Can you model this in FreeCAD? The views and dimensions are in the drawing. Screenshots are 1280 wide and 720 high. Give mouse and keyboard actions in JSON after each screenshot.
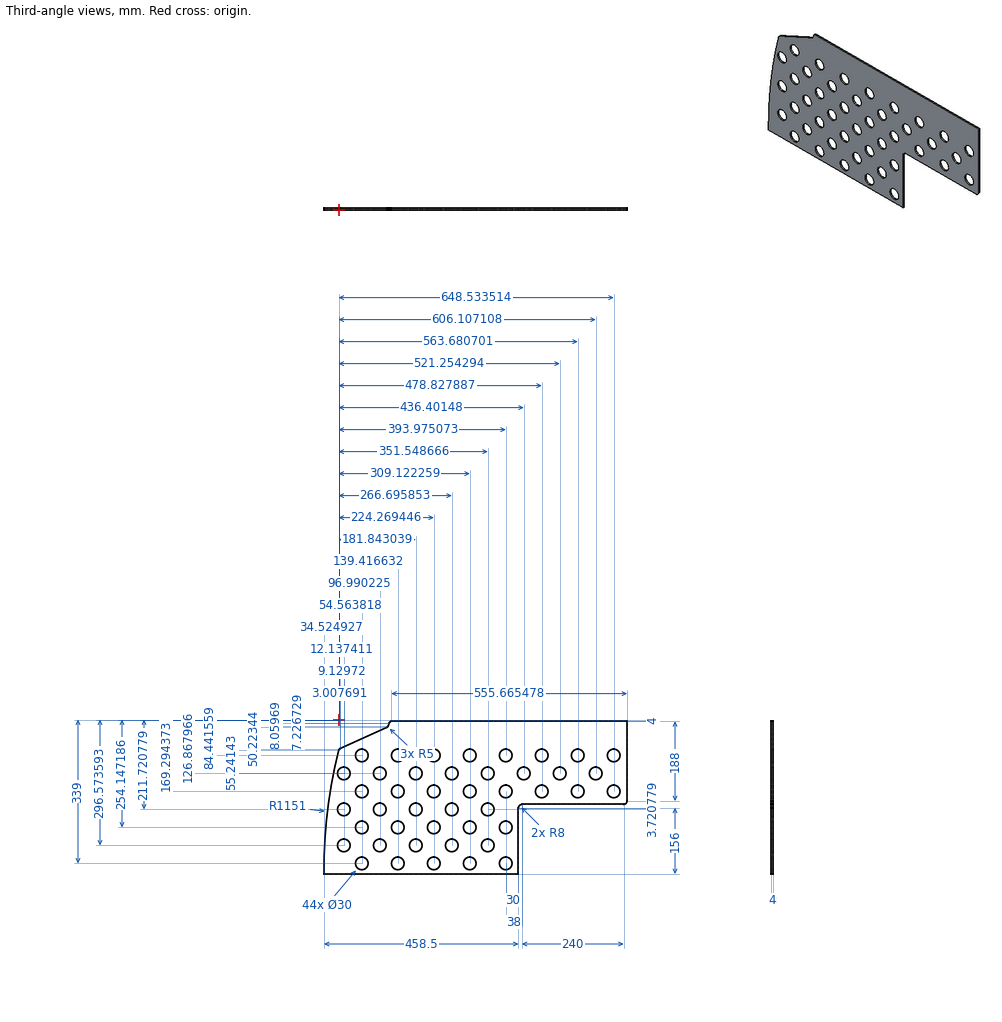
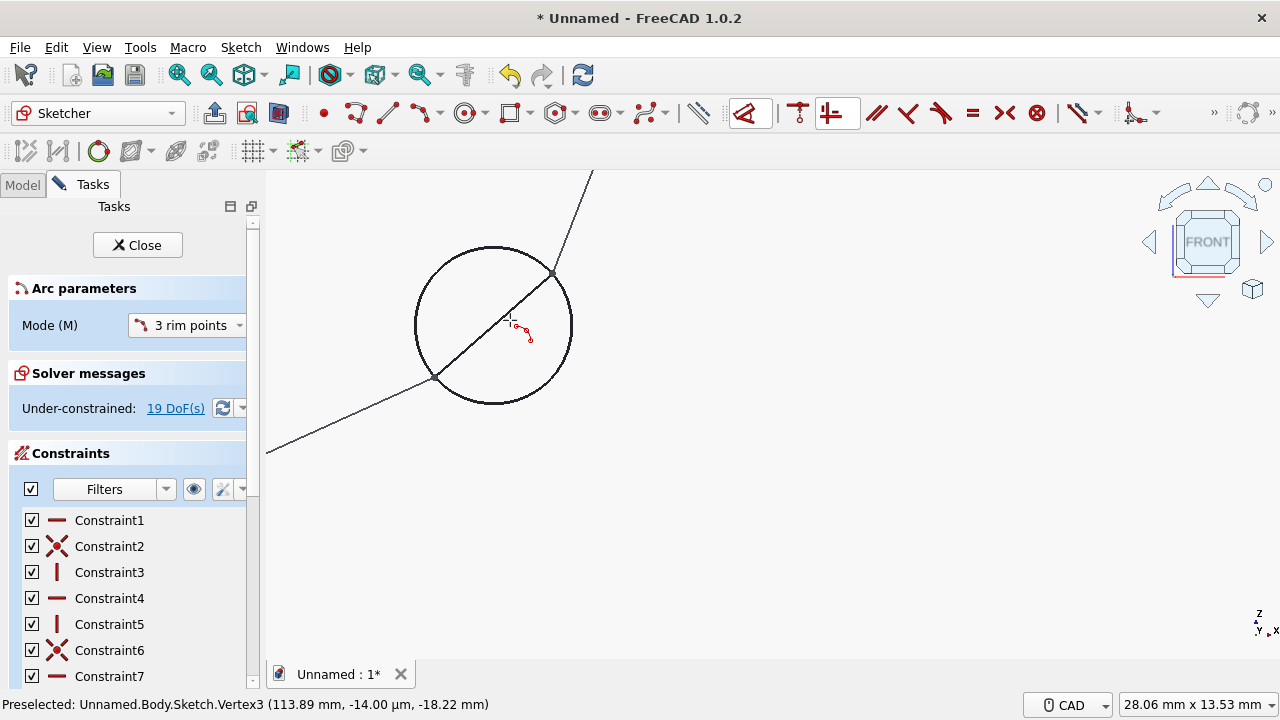
{"action": "left_click", "coordinate": [508, 321]}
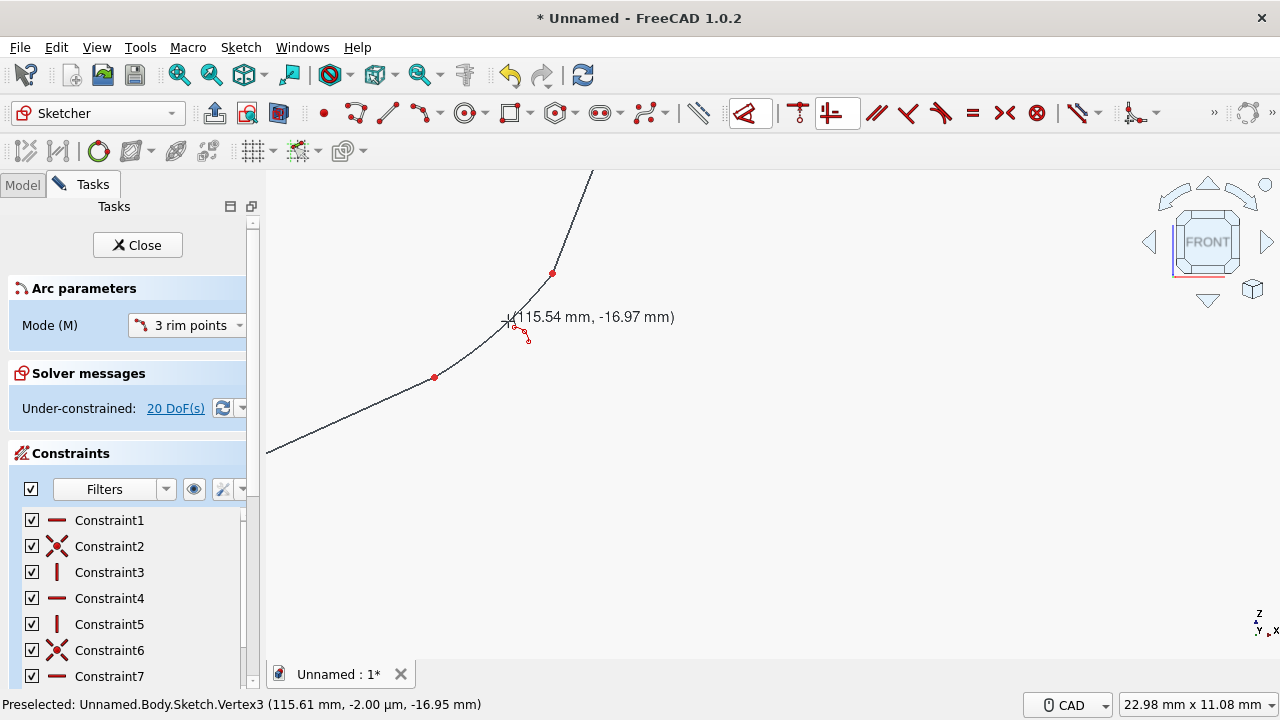
{"action": "scroll", "coordinate": [704, 414], "scroll_direction": "down", "scroll_amount": 15}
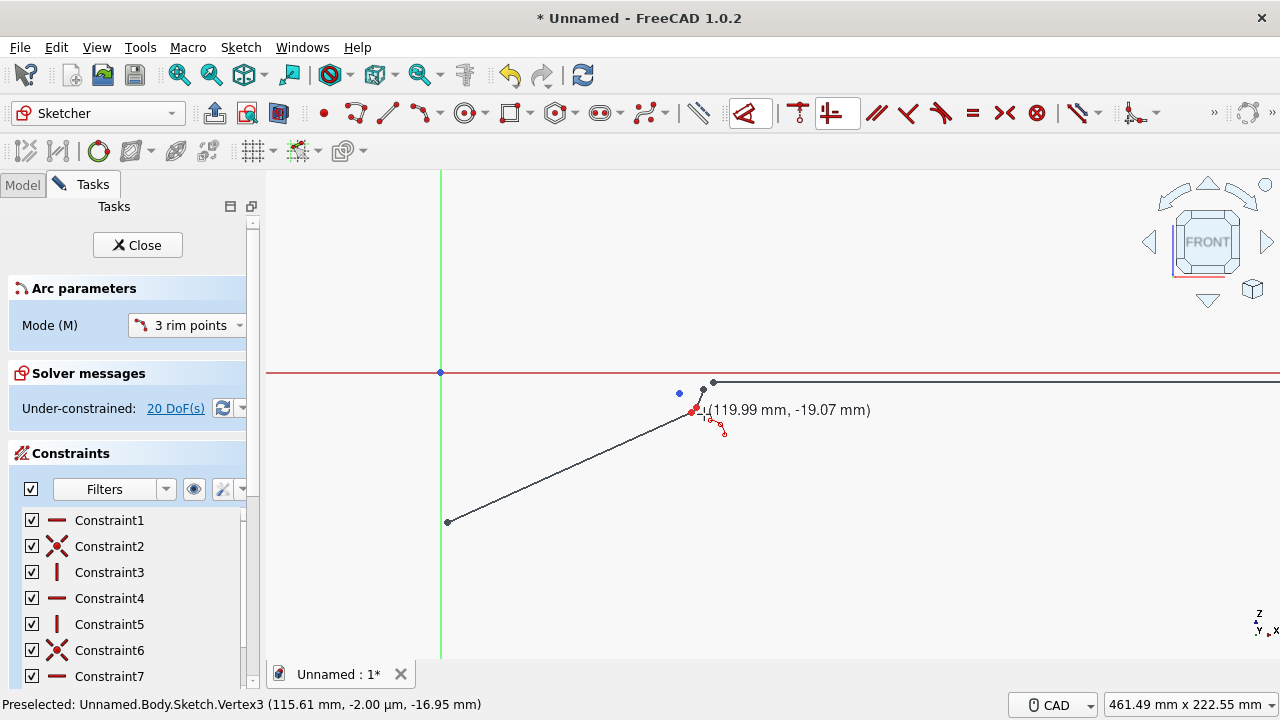
{"action": "scroll", "coordinate": [445, 206], "scroll_direction": "down", "scroll_amount": 5}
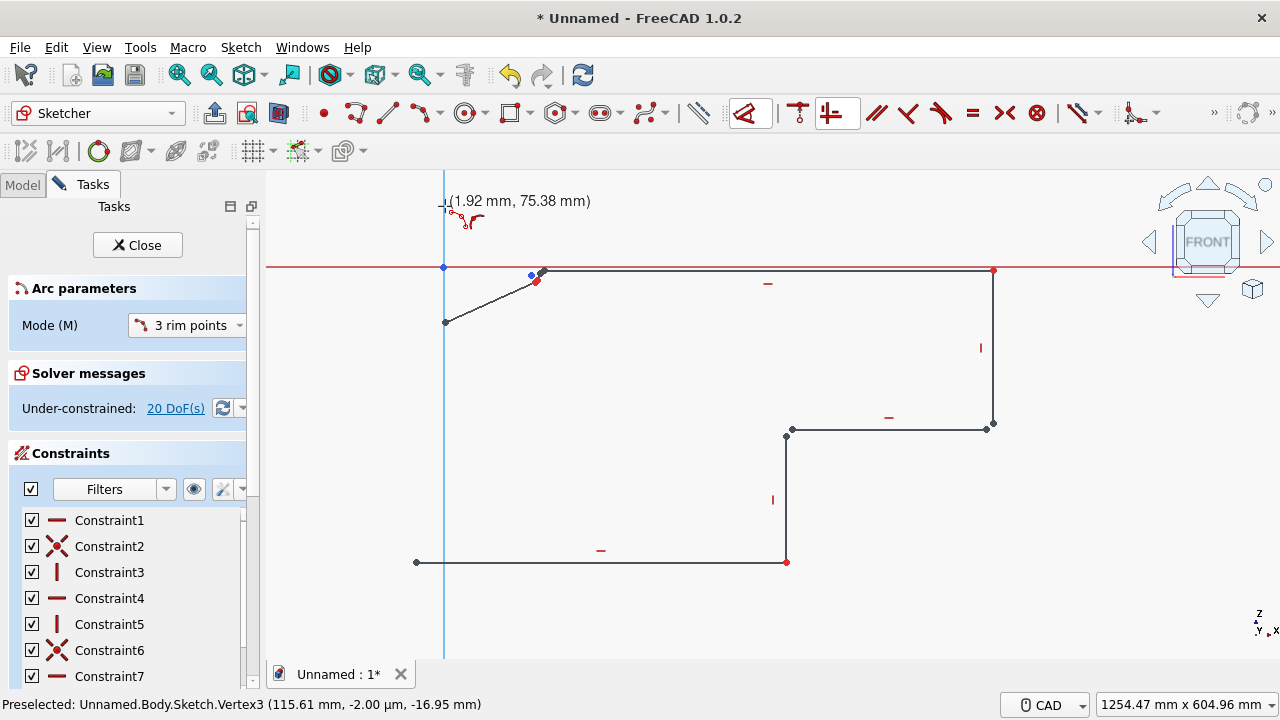
{"action": "scroll", "coordinate": [446, 323], "scroll_direction": "up", "scroll_amount": 10}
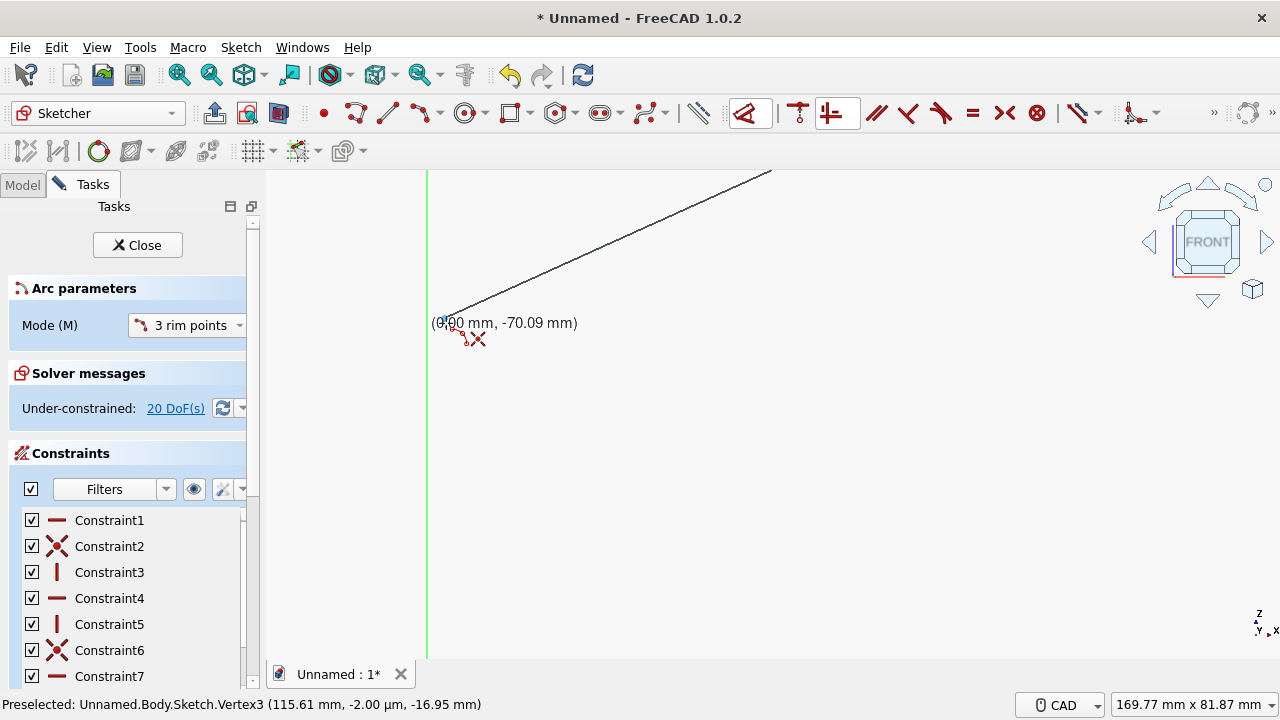
{"action": "left_click", "coordinate": [444, 318]}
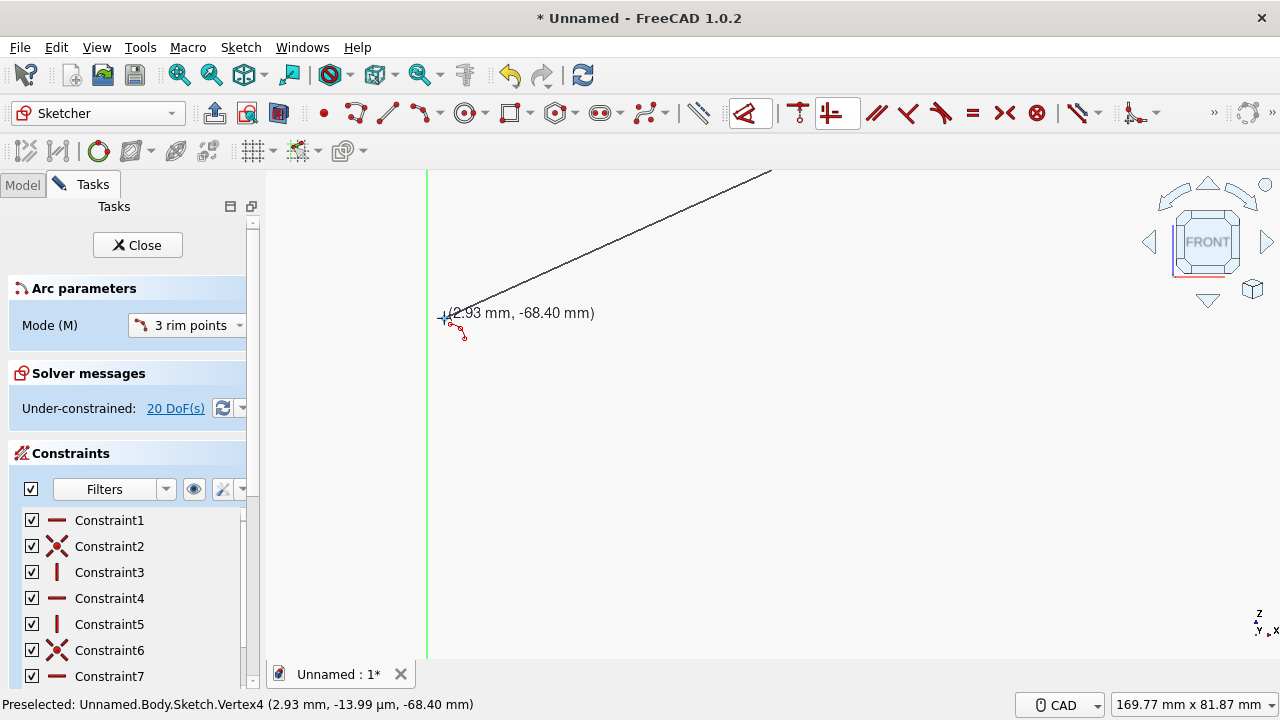
{"action": "scroll", "coordinate": [428, 338], "scroll_direction": "up", "scroll_amount": 13}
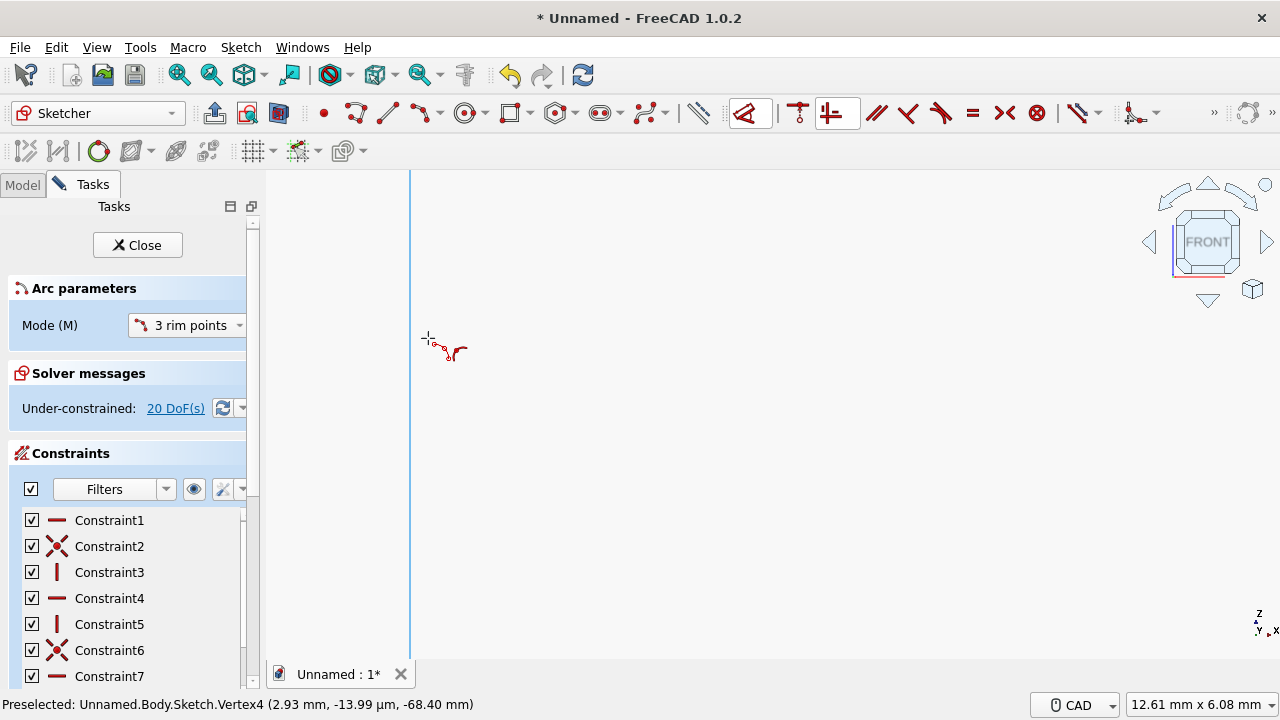
{"action": "left_click", "coordinate": [428, 328]}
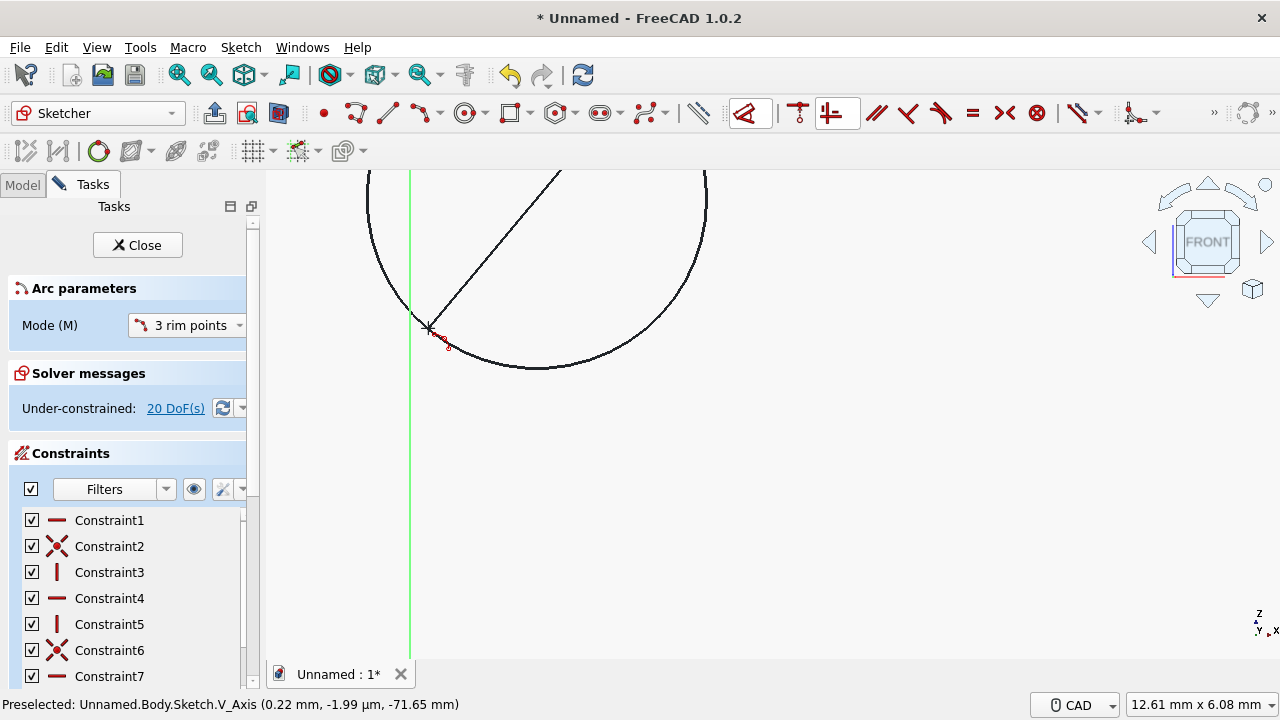
{"action": "scroll", "coordinate": [704, 414], "scroll_direction": "down", "scroll_amount": 15}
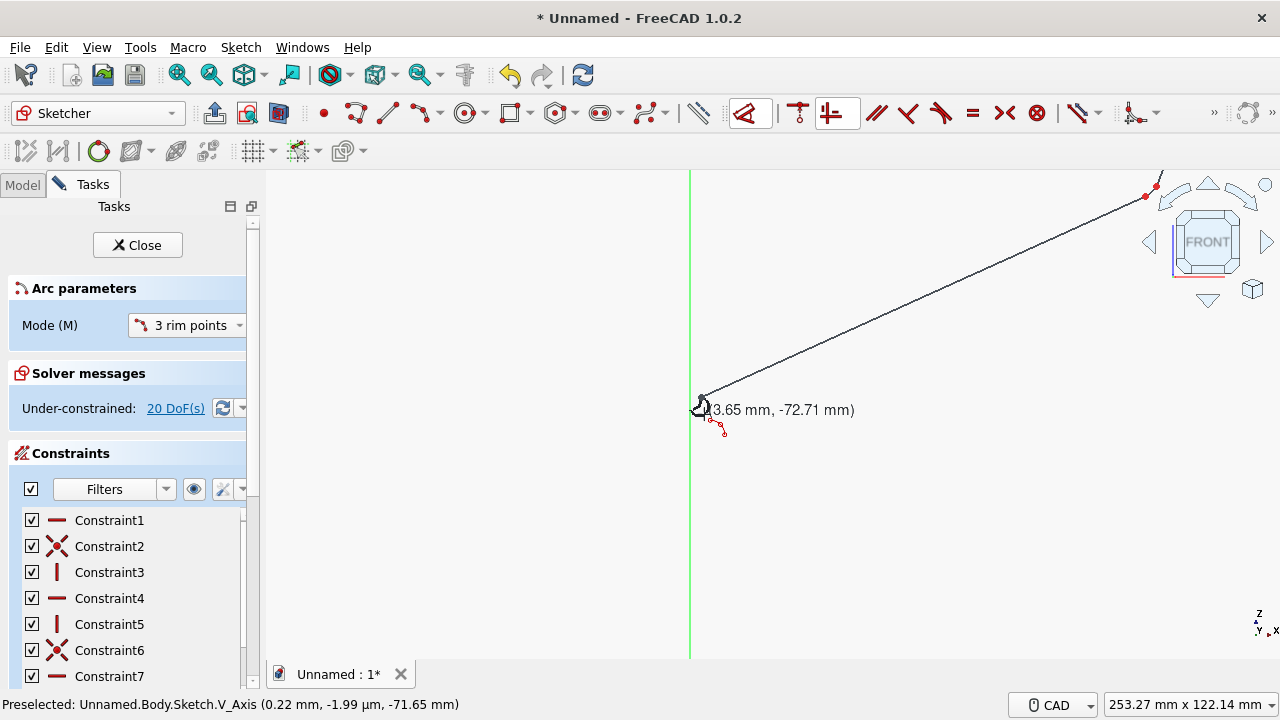
{"action": "scroll", "coordinate": [381, 304], "scroll_direction": "down", "scroll_amount": 8}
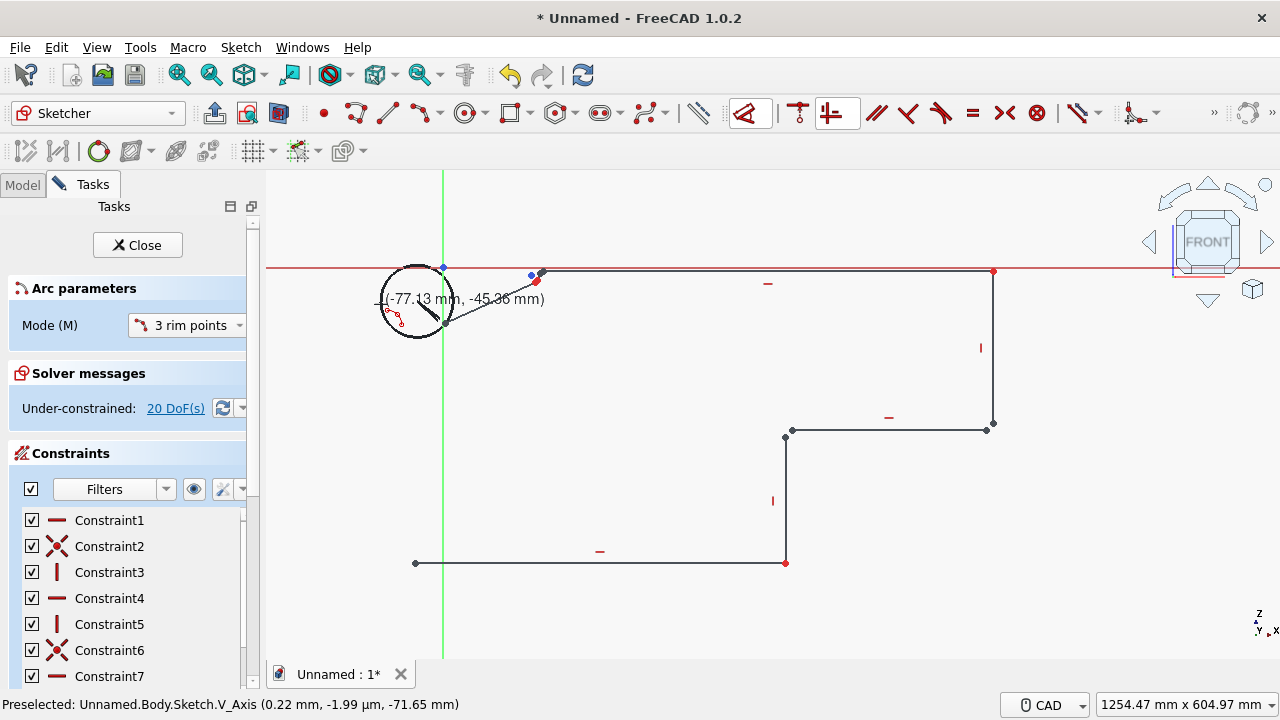
{"action": "scroll", "coordinate": [444, 324], "scroll_direction": "up", "scroll_amount": 19}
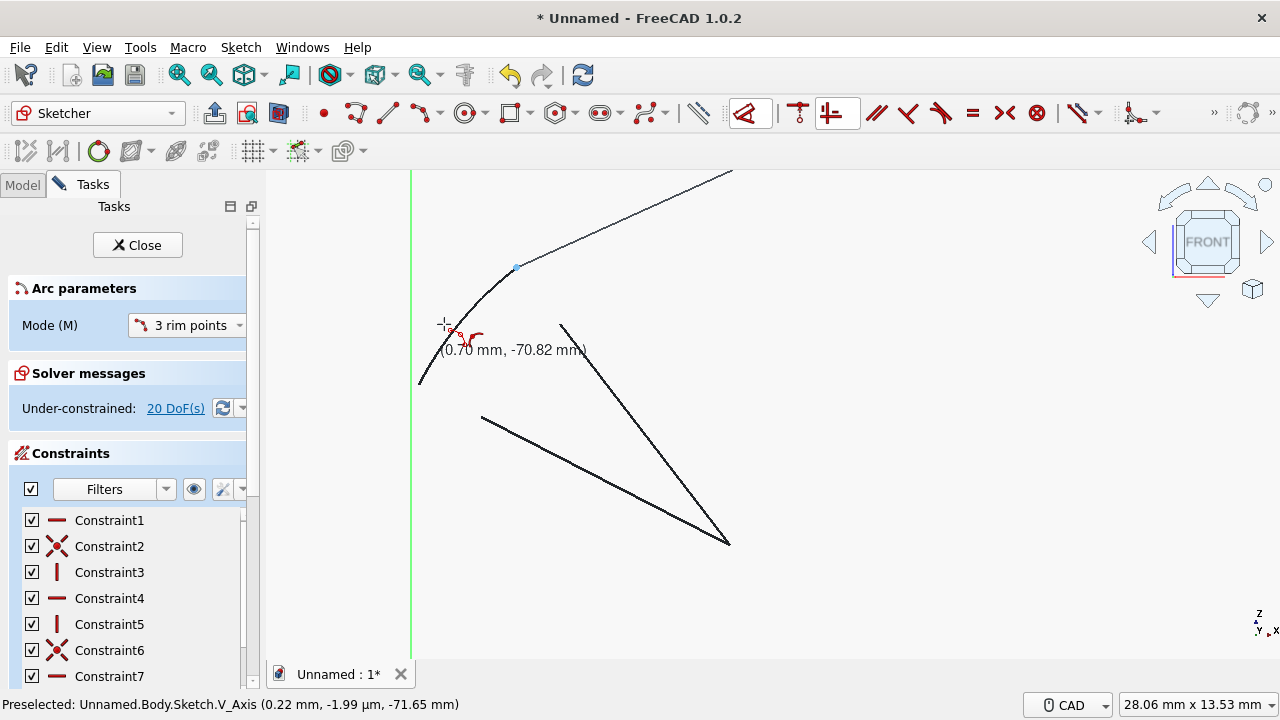
{"action": "left_click", "coordinate": [455, 312]}